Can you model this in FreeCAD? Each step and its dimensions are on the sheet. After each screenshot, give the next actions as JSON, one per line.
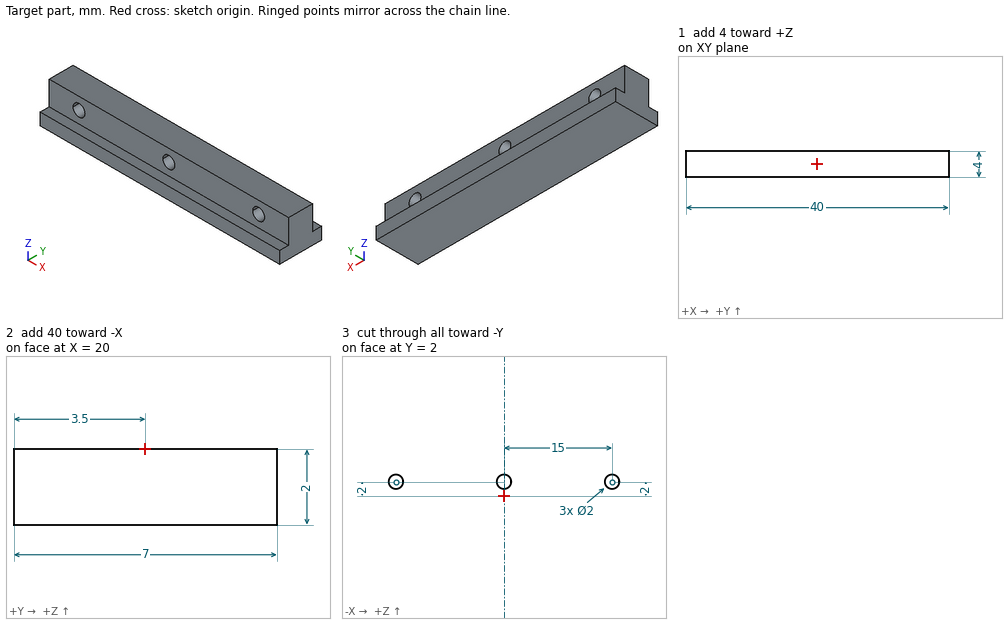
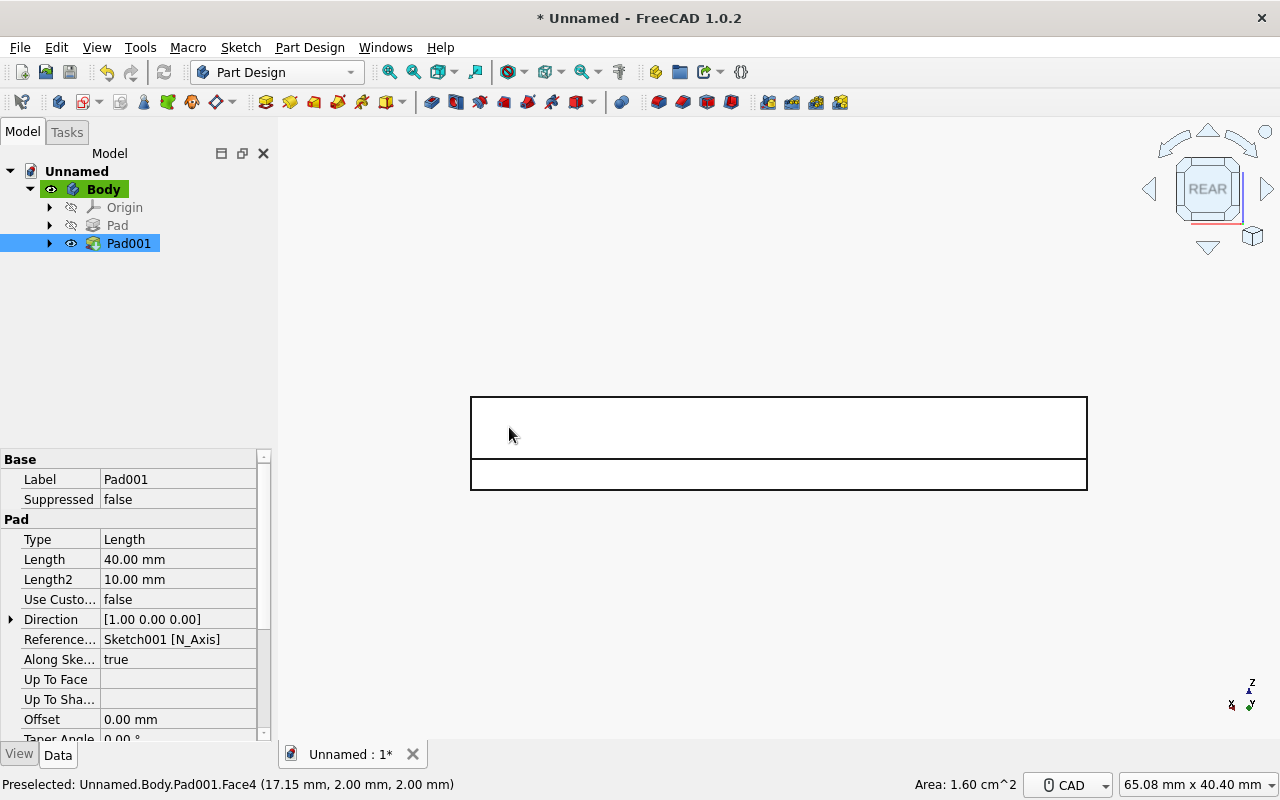
{"action": "left_click", "coordinate": [84, 102]}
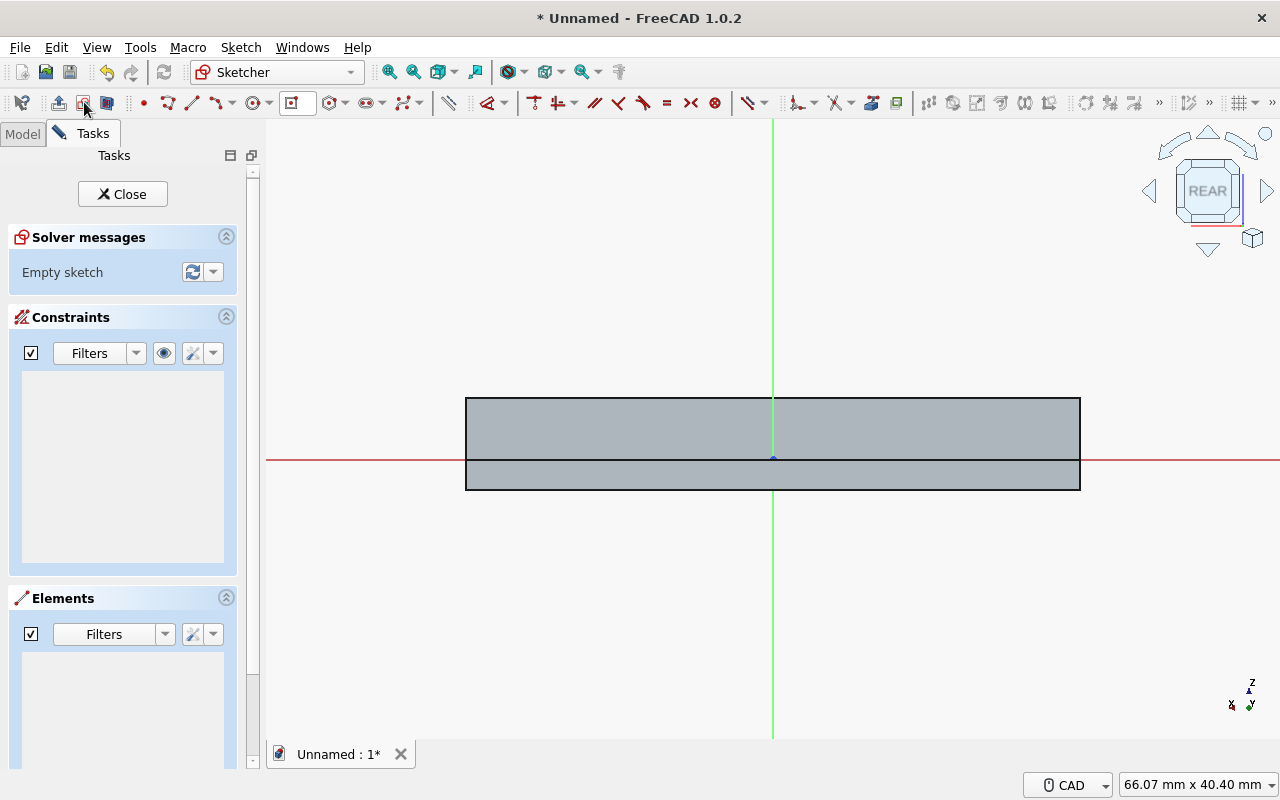
{"action": "key", "text": "g c"}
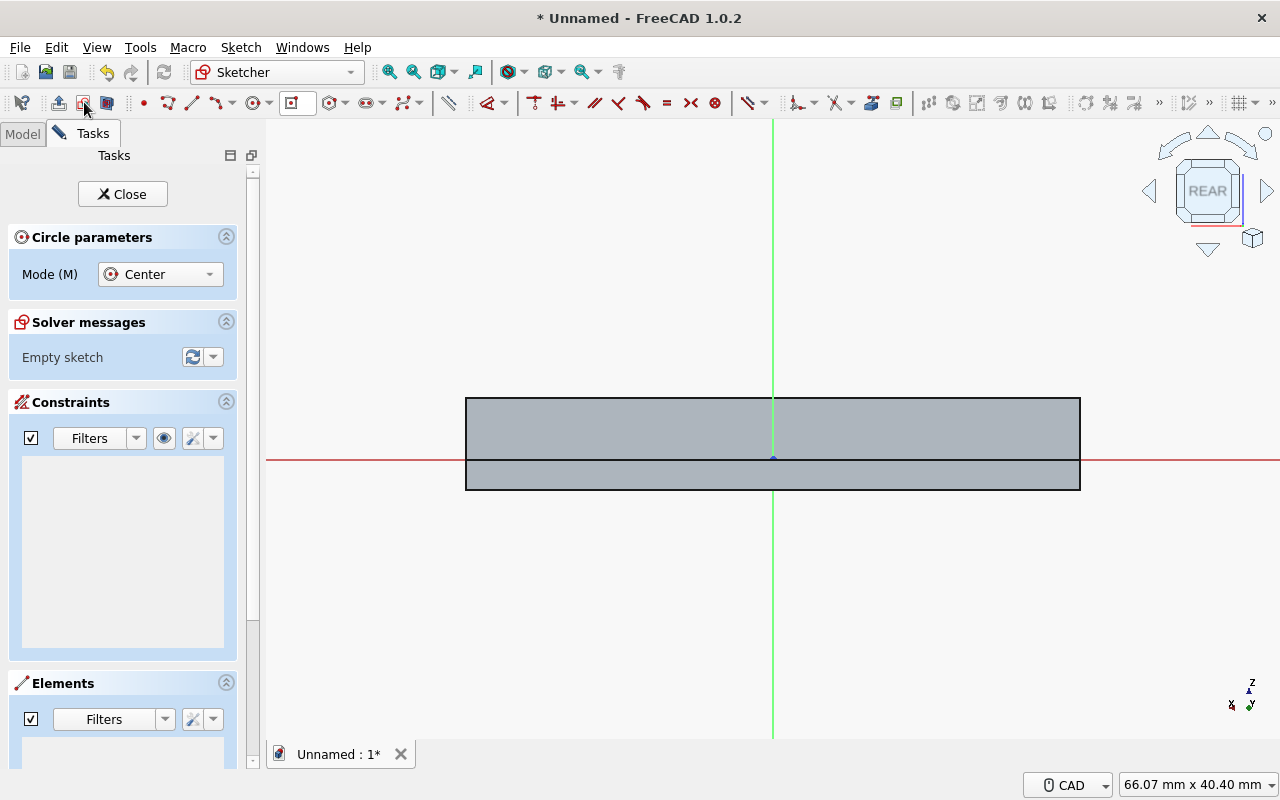
{"action": "scroll", "coordinate": [1003, 429], "scroll_direction": "up", "scroll_amount": 2}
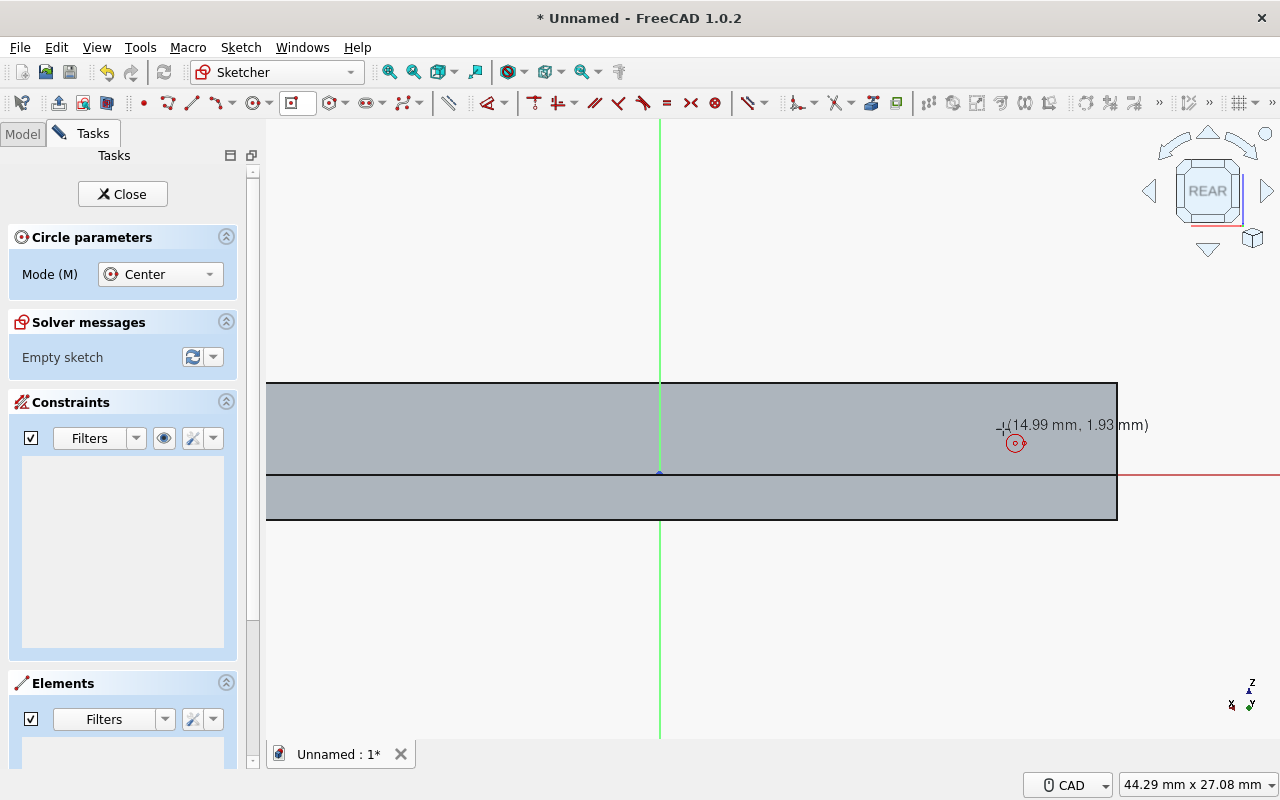
{"action": "left_click", "coordinate": [1003, 429]}
{"action": "mouse_move", "coordinate": [1019, 413]}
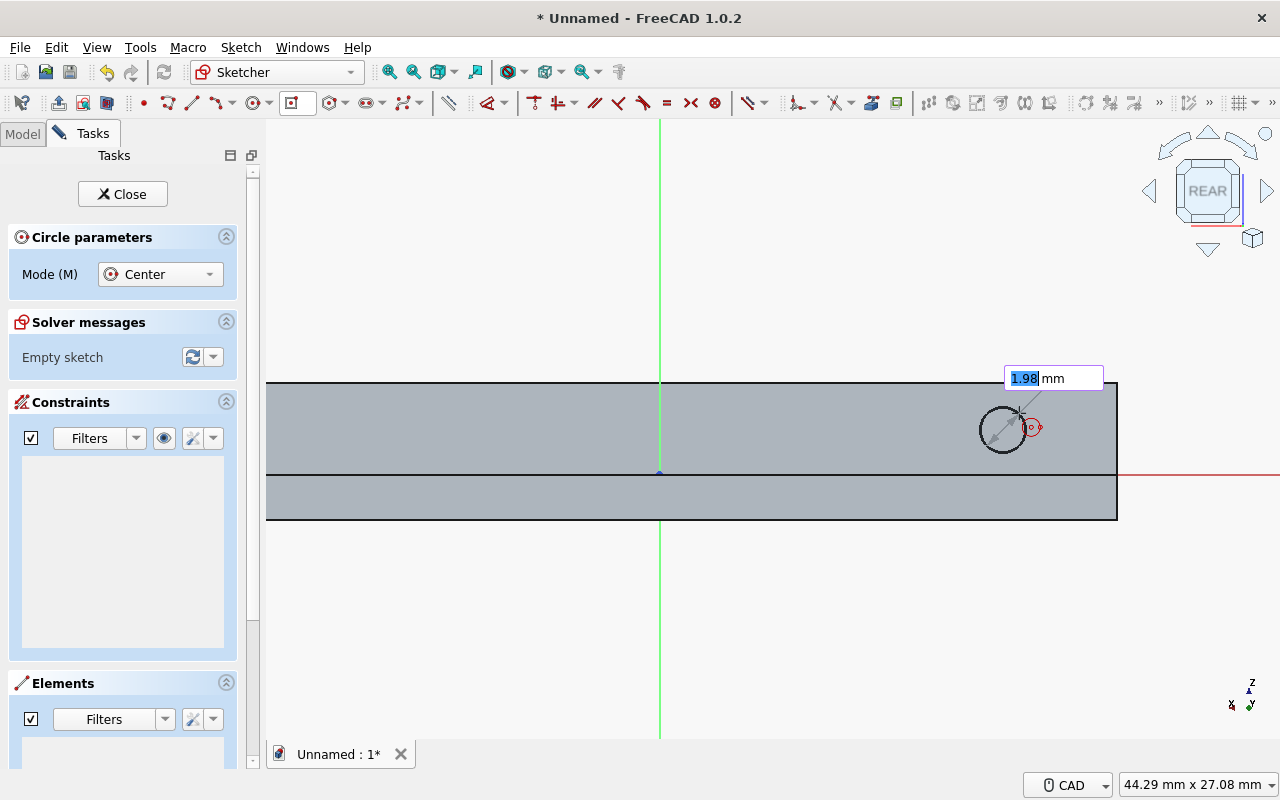
{"action": "type", "text": "2"}
{"action": "key", "text": "Return"}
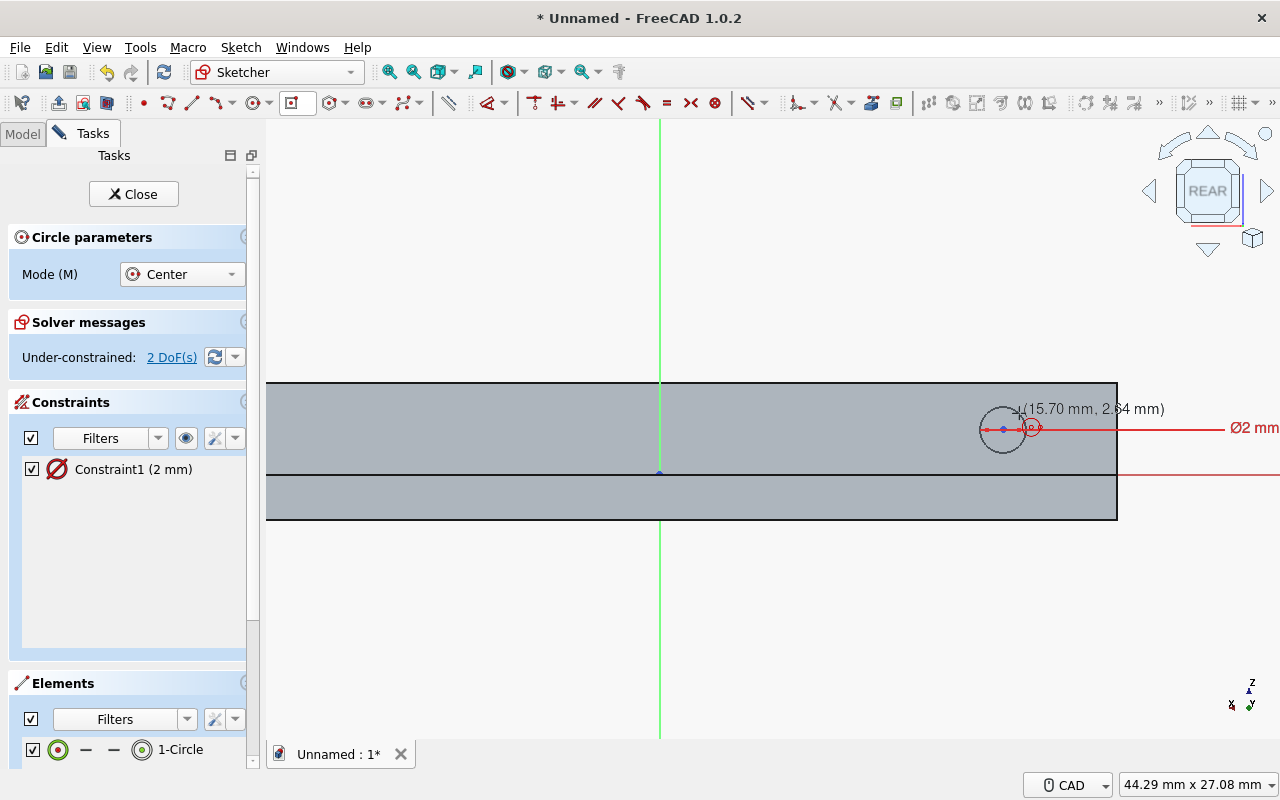
{"action": "left_click", "coordinate": [660, 429]}
{"action": "mouse_move", "coordinate": [676, 413]}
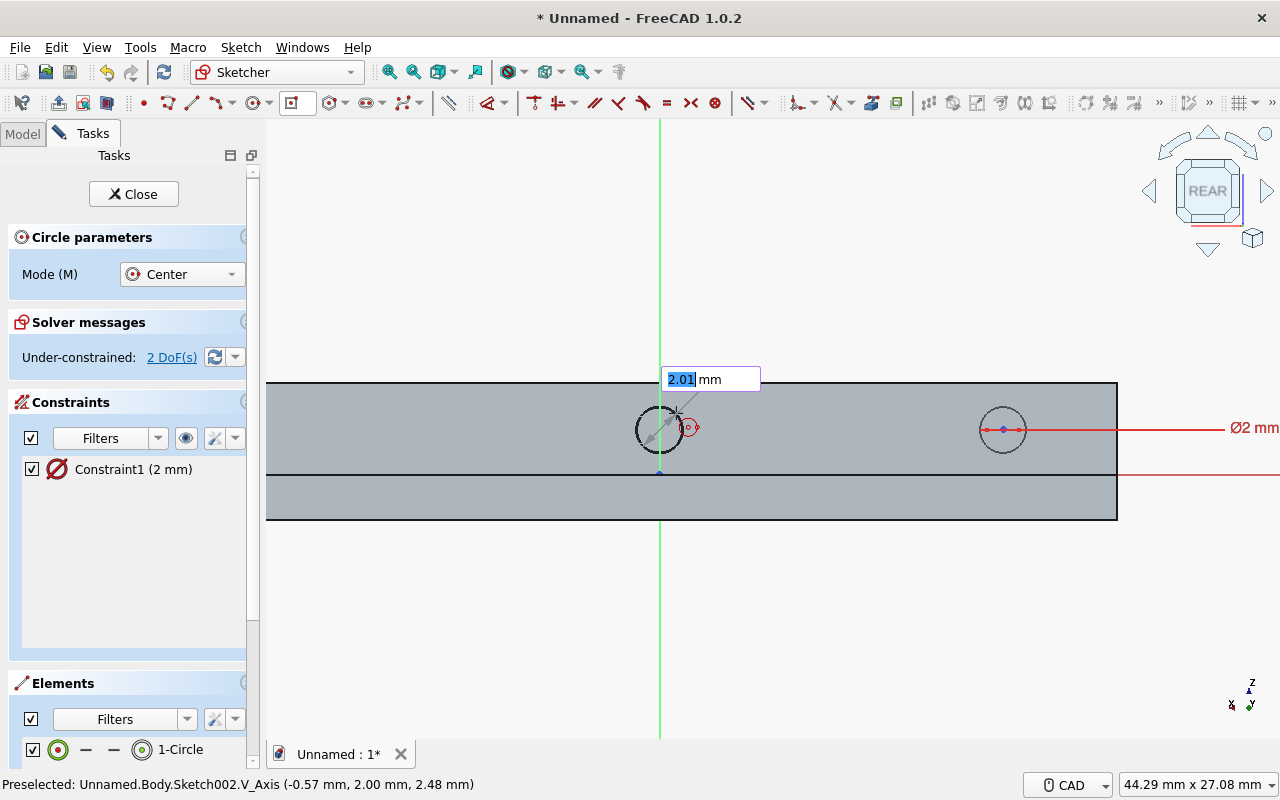
{"action": "type", "text": "2"}
{"action": "key", "text": "Return"}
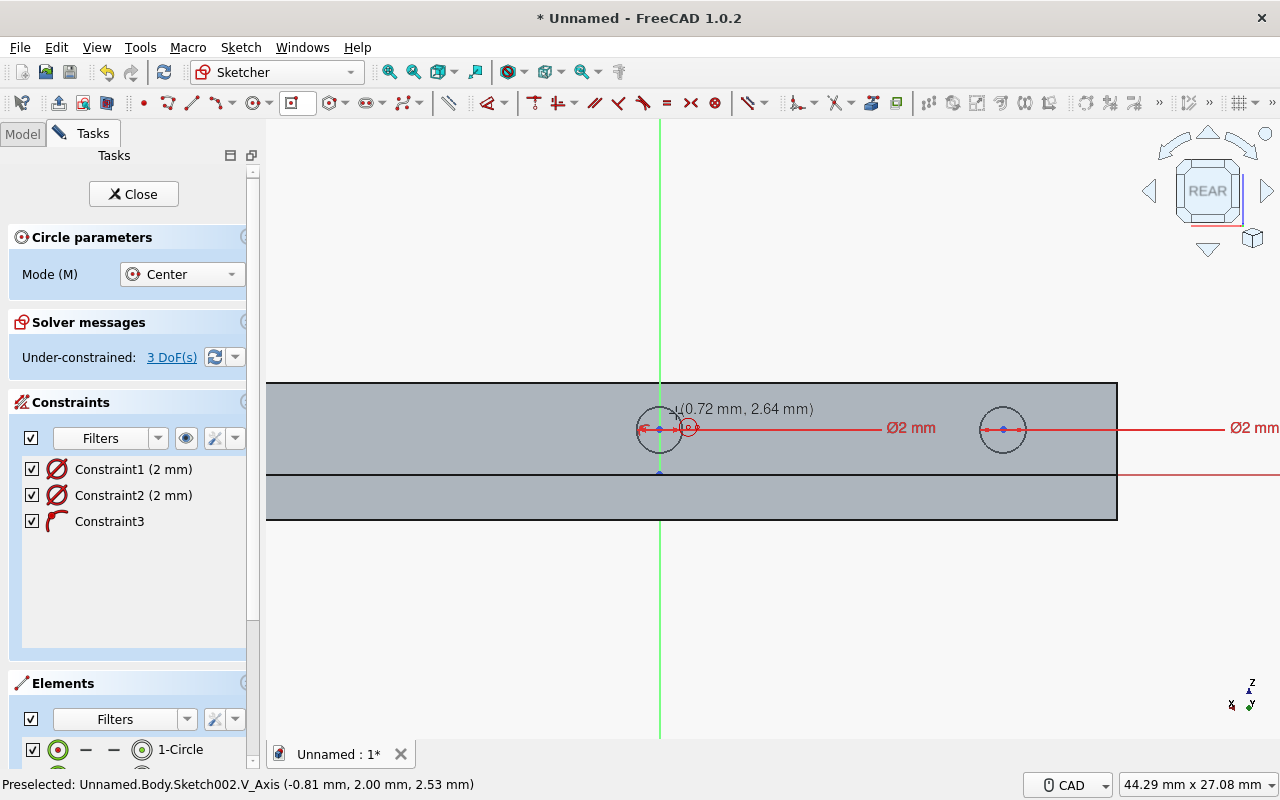
{"action": "left_click", "coordinate": [316, 429]}
{"action": "mouse_move", "coordinate": [332, 413]}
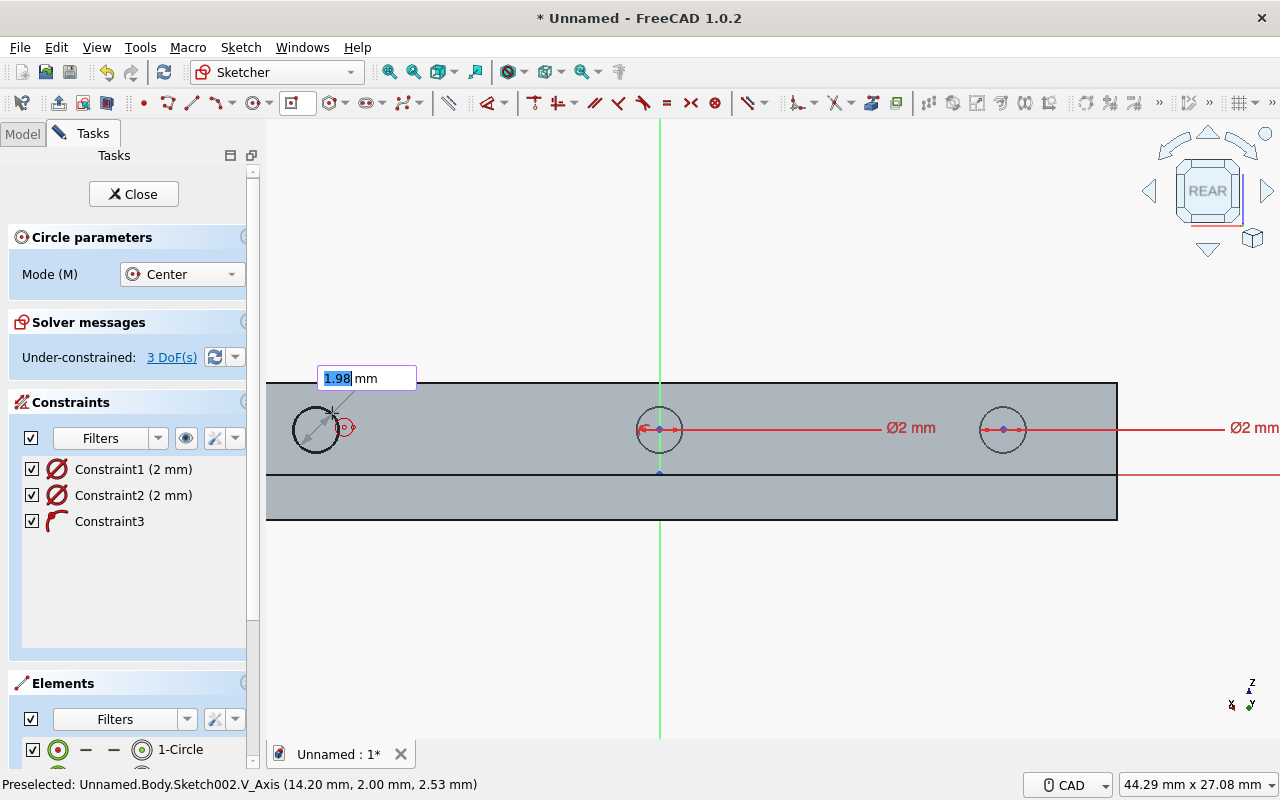
{"action": "type", "text": "2"}
{"action": "key", "text": "Return"}
{"action": "key", "text": "Escape"}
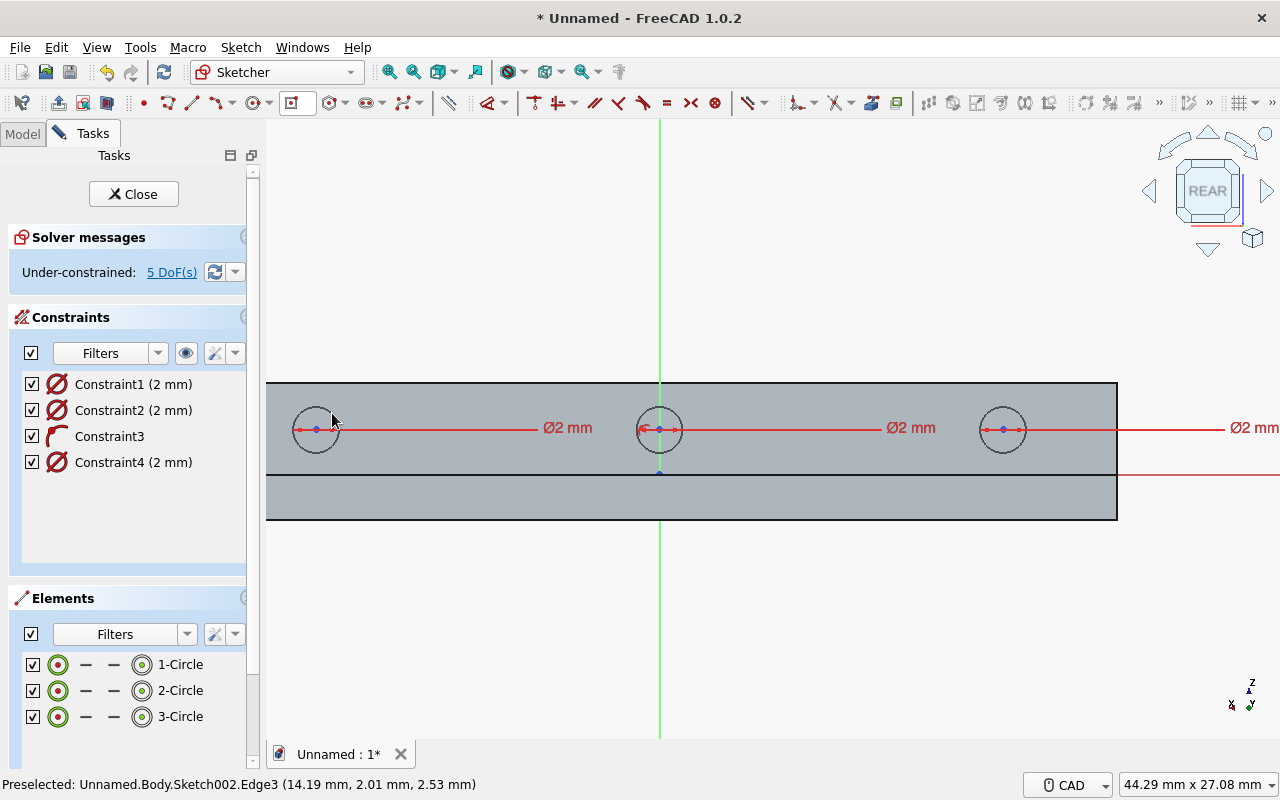
{"action": "left_click", "coordinate": [1003, 430]}